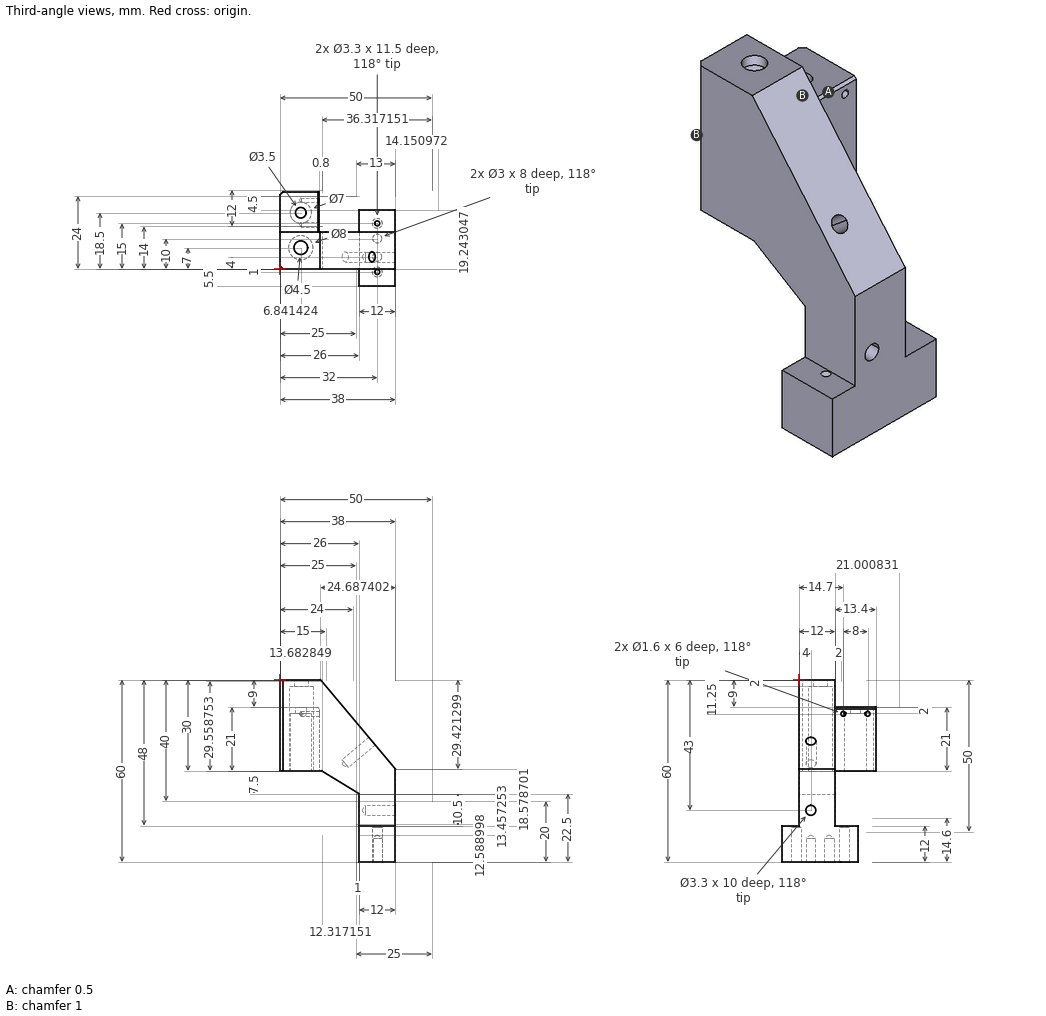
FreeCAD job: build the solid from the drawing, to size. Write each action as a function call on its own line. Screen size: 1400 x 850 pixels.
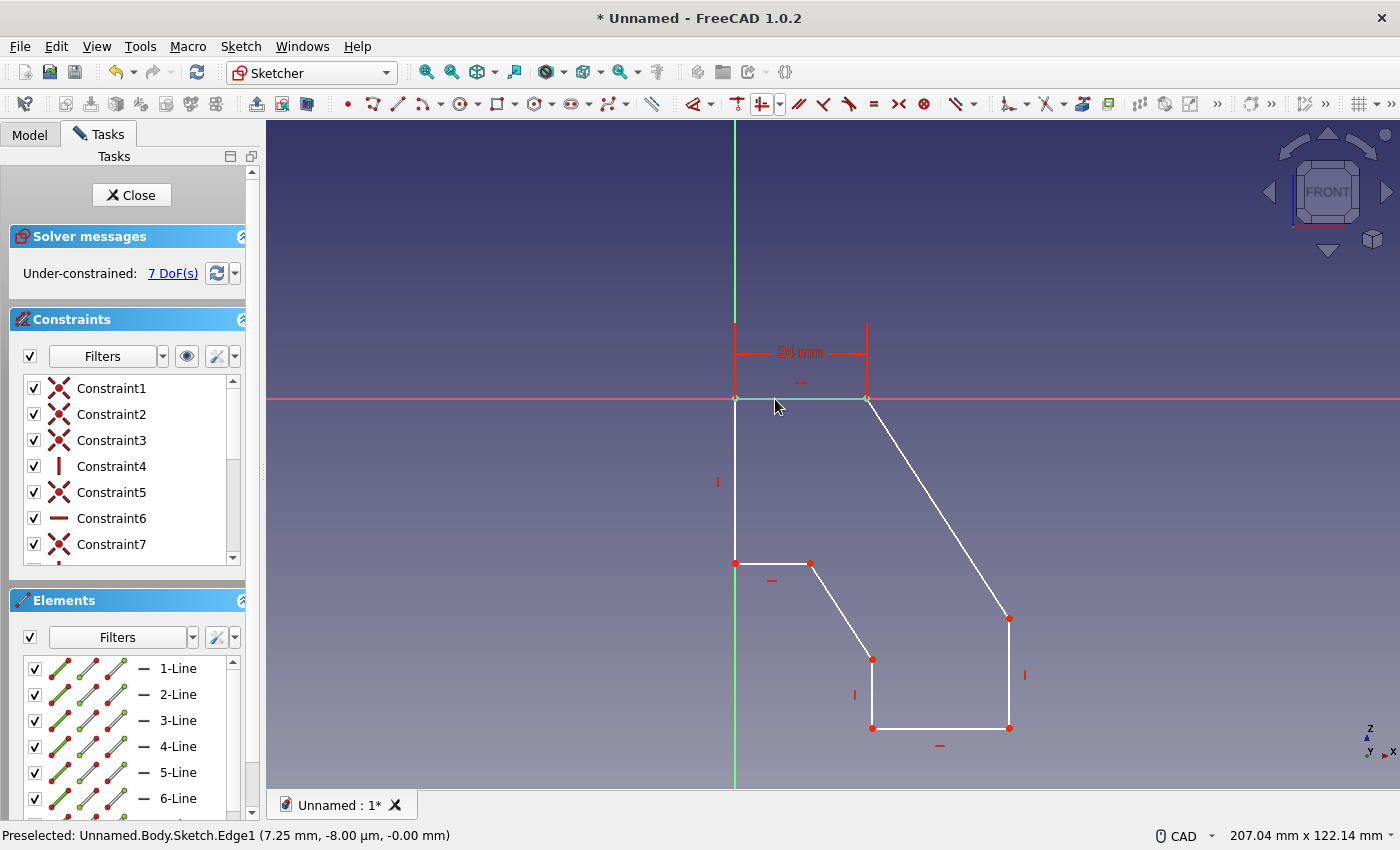
click(1009, 652)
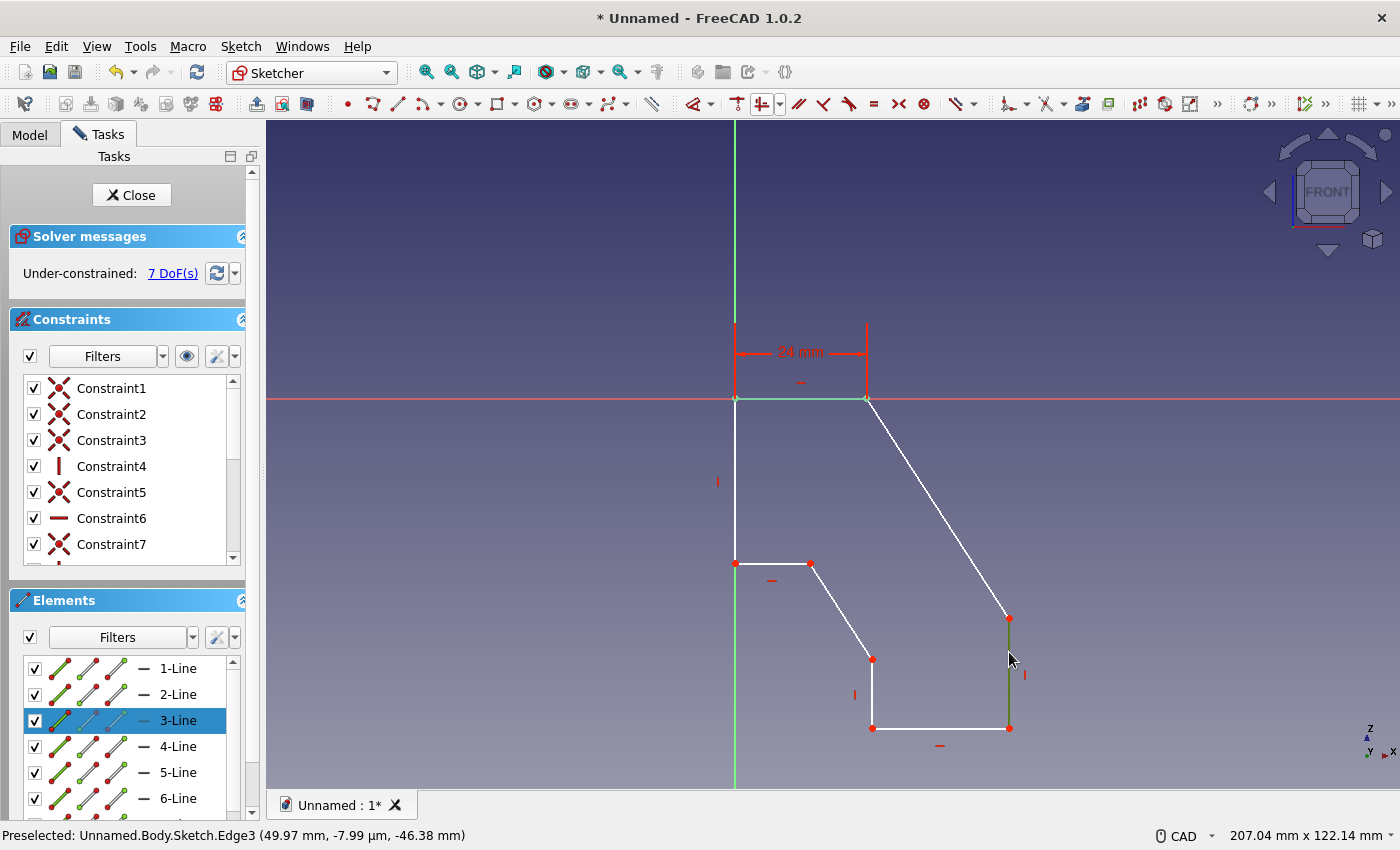
click(710, 104)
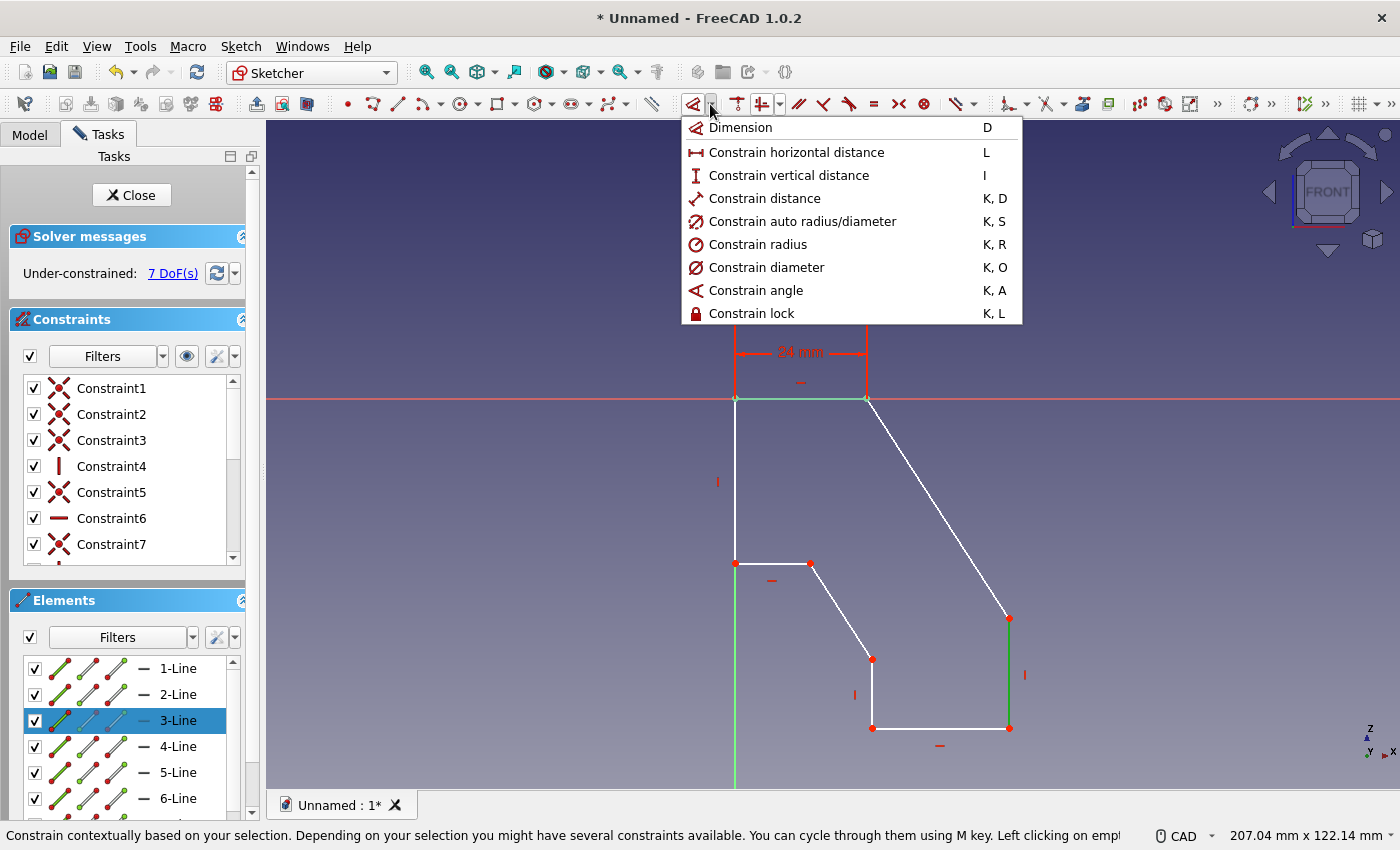
click(852, 176)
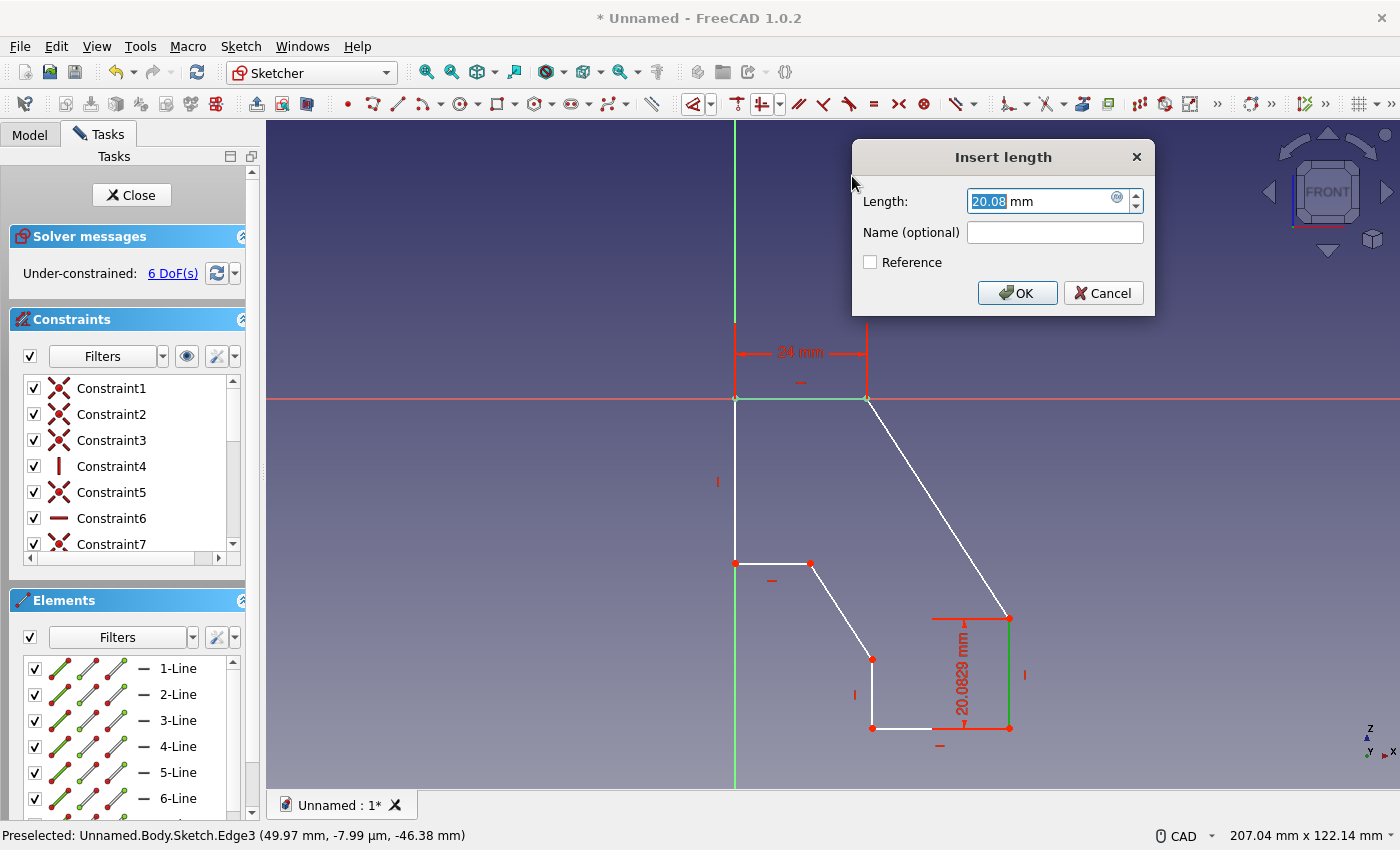
text(20)
key(Return)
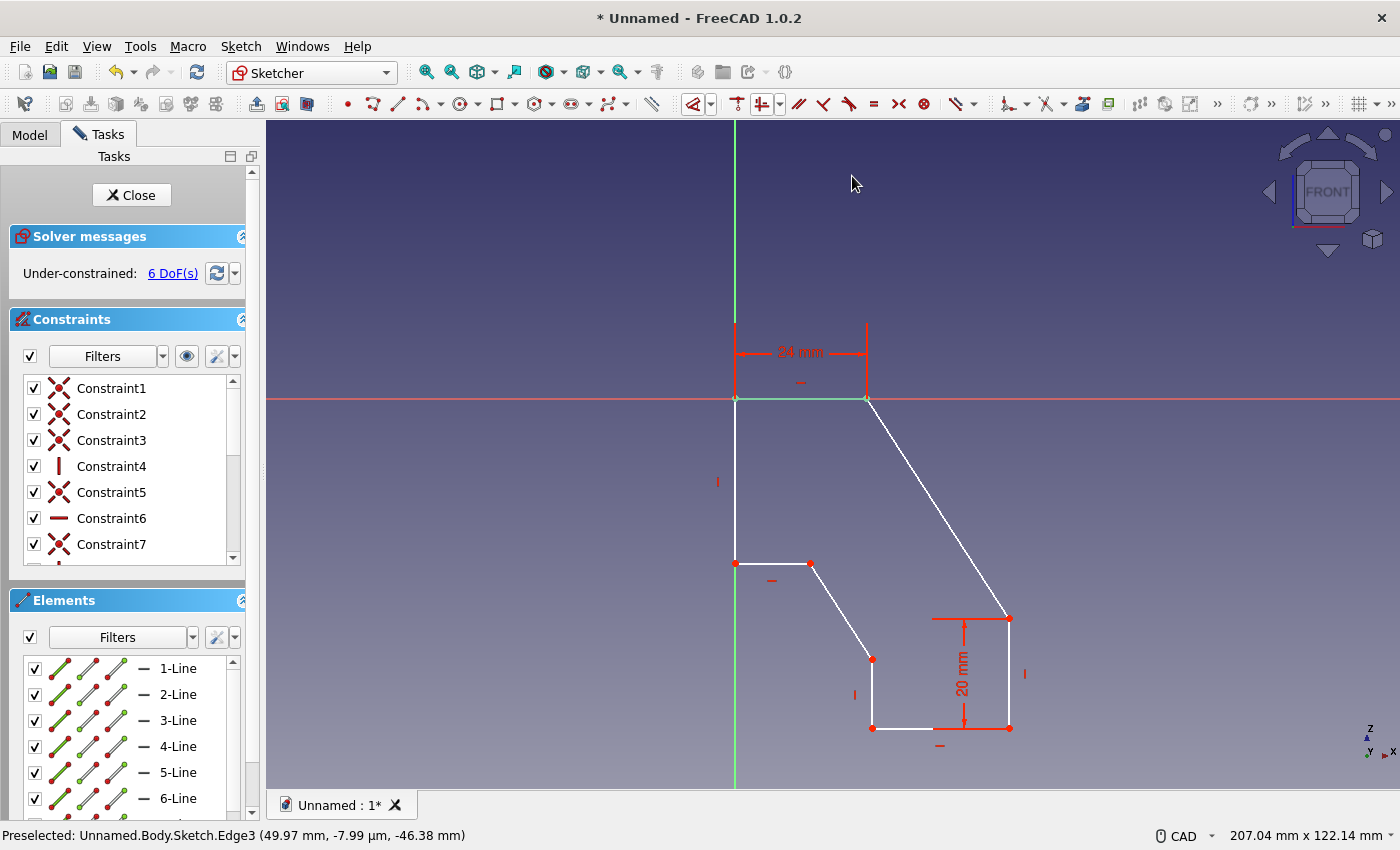
click(968, 729)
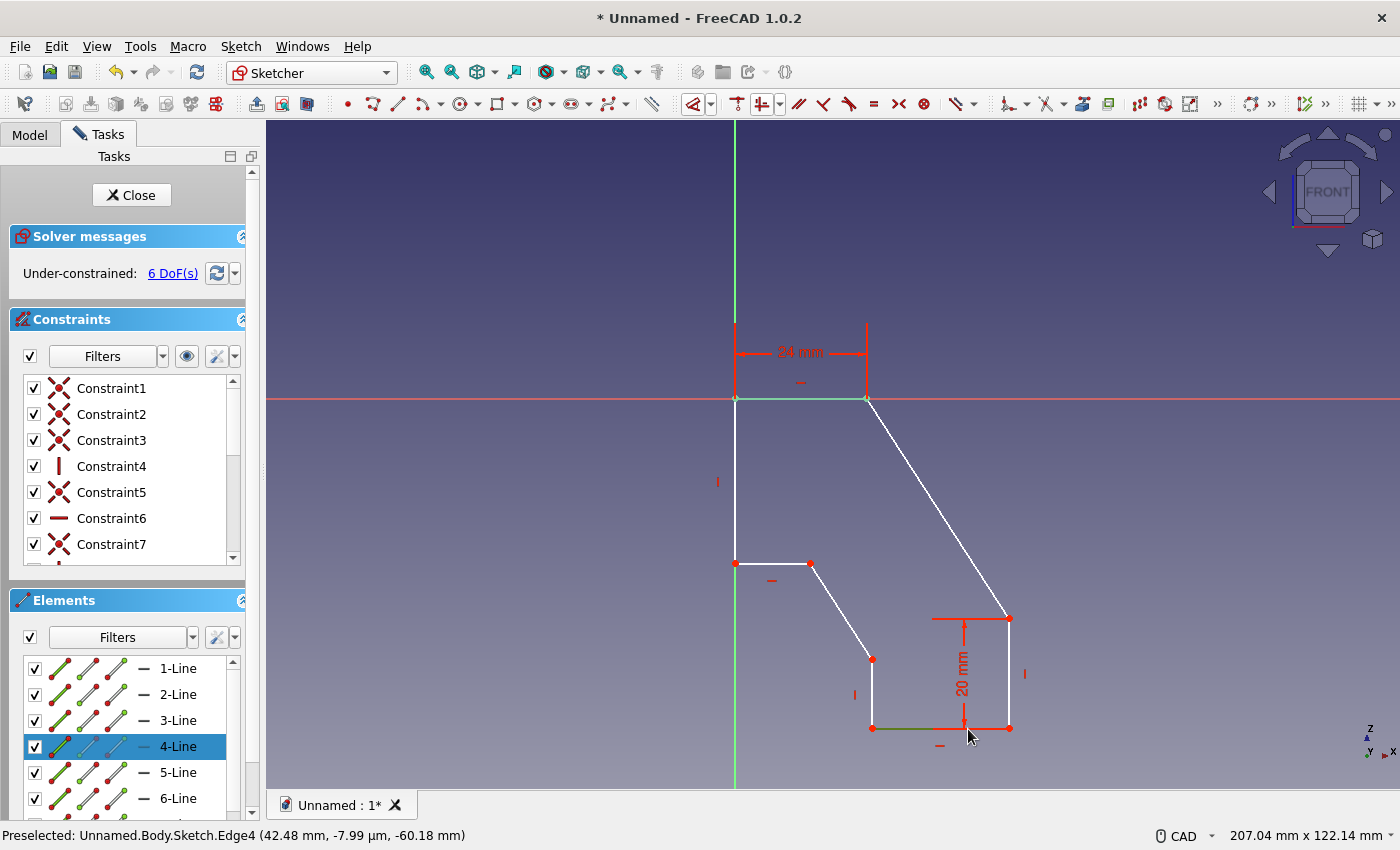
click(710, 104)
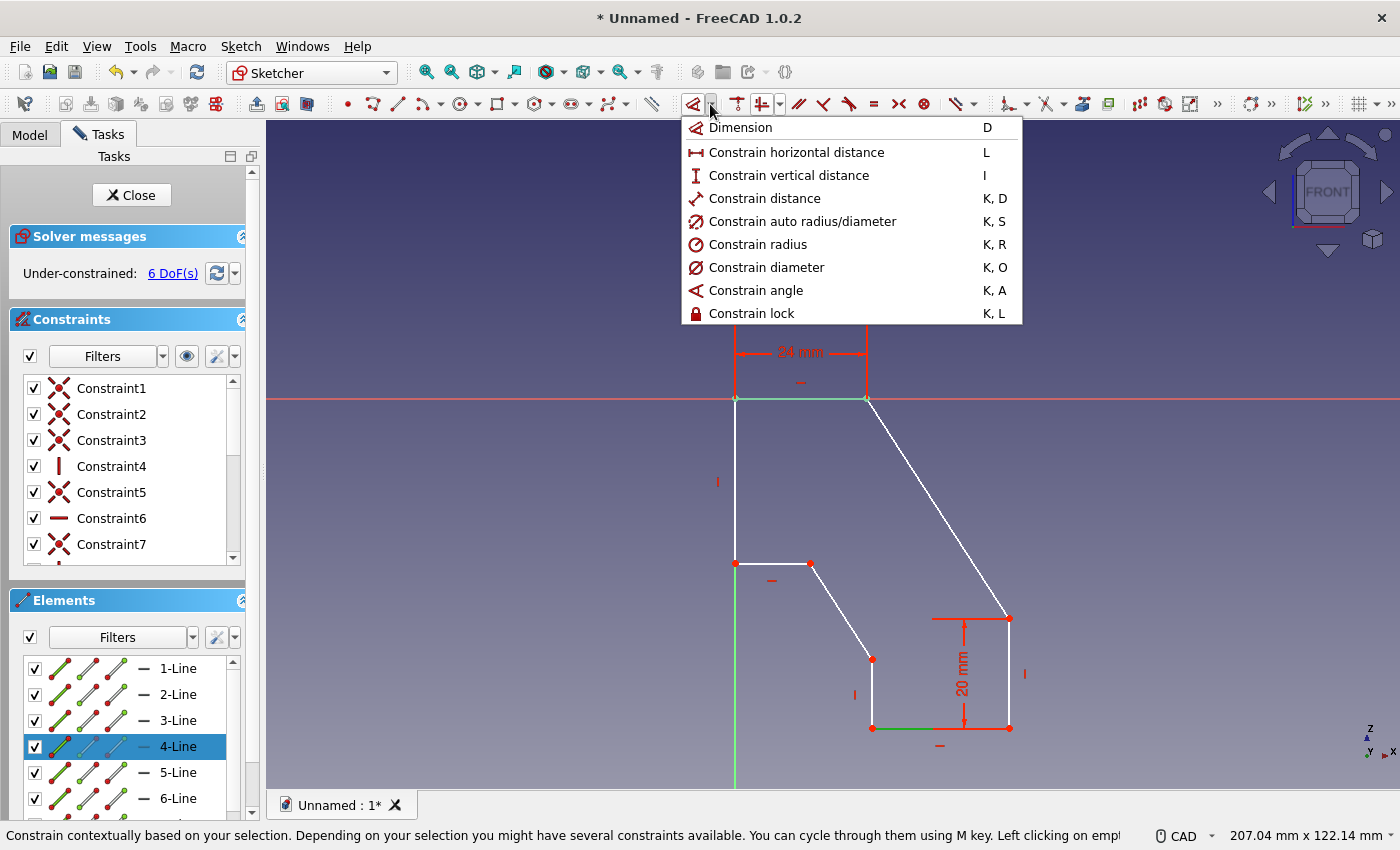
click(852, 152)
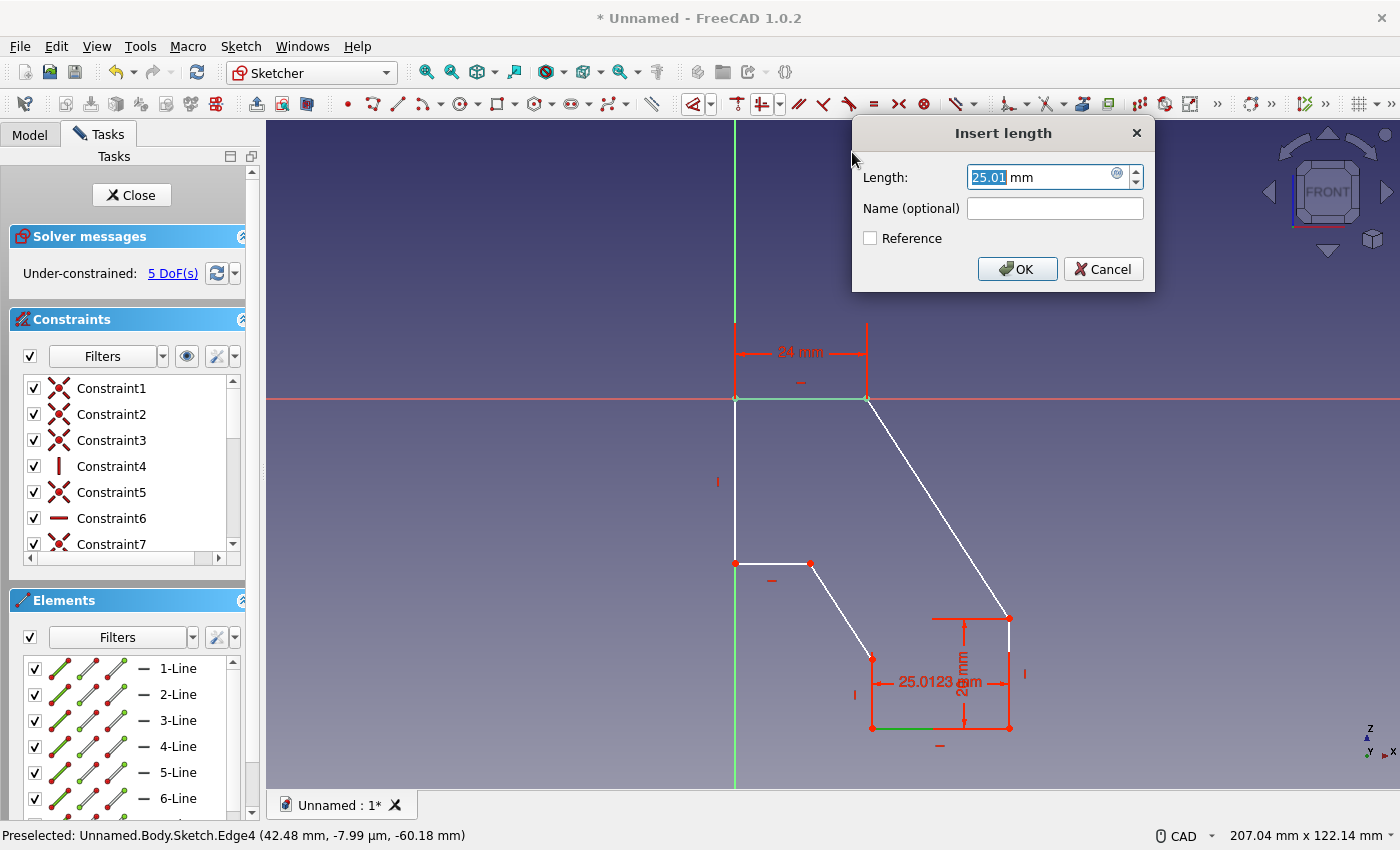
text(25)
key(Return)